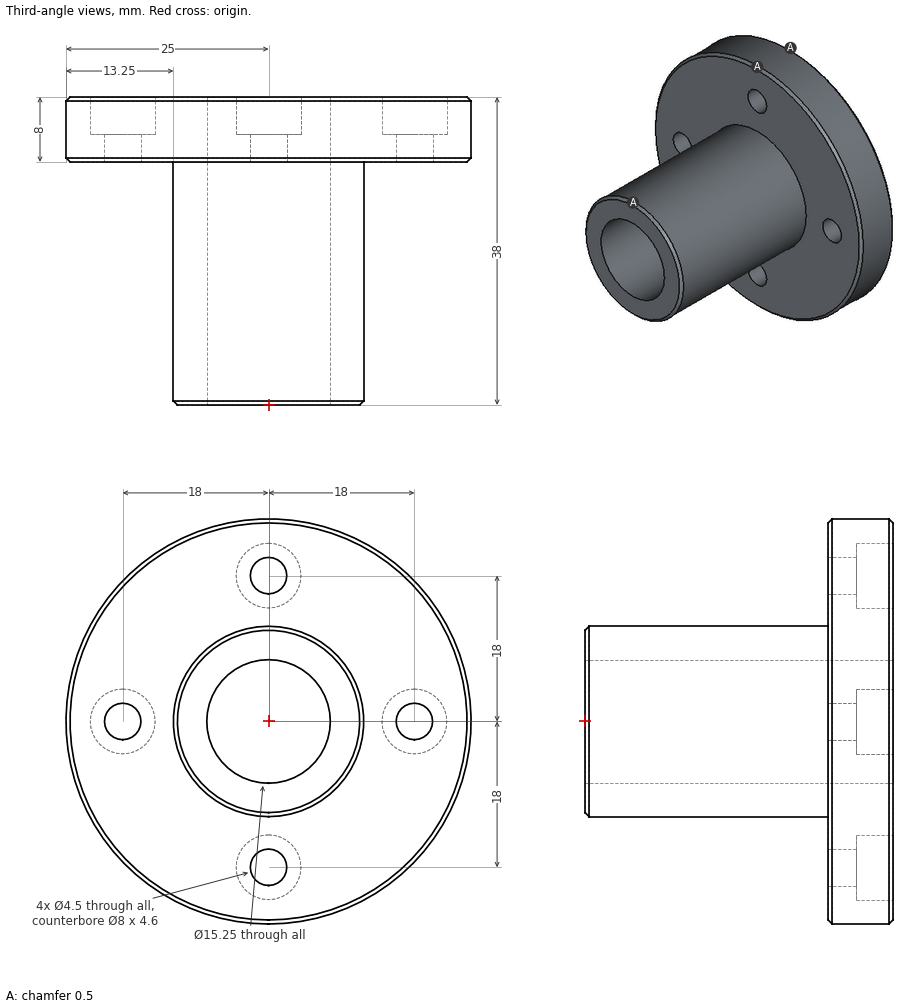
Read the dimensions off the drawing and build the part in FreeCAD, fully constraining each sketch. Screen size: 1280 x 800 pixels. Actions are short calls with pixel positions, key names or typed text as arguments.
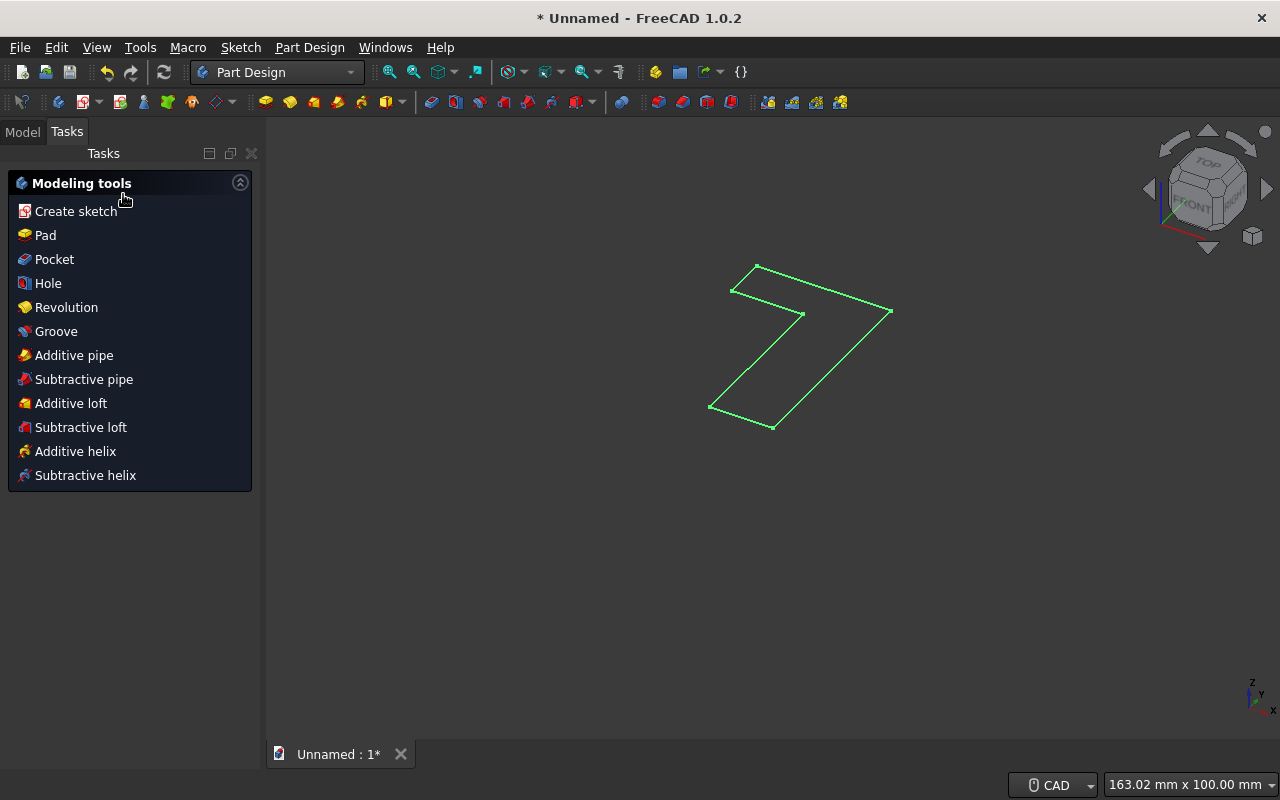
click(290, 102)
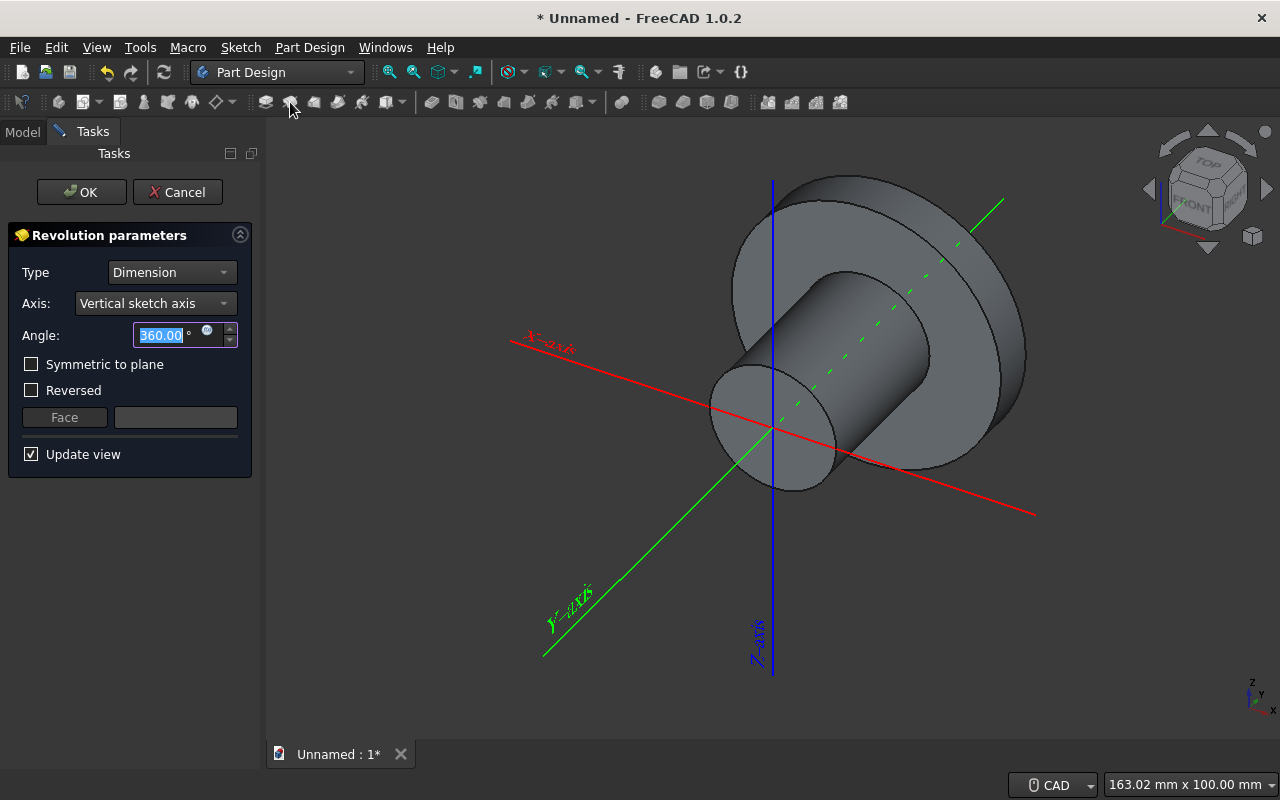
click(82, 192)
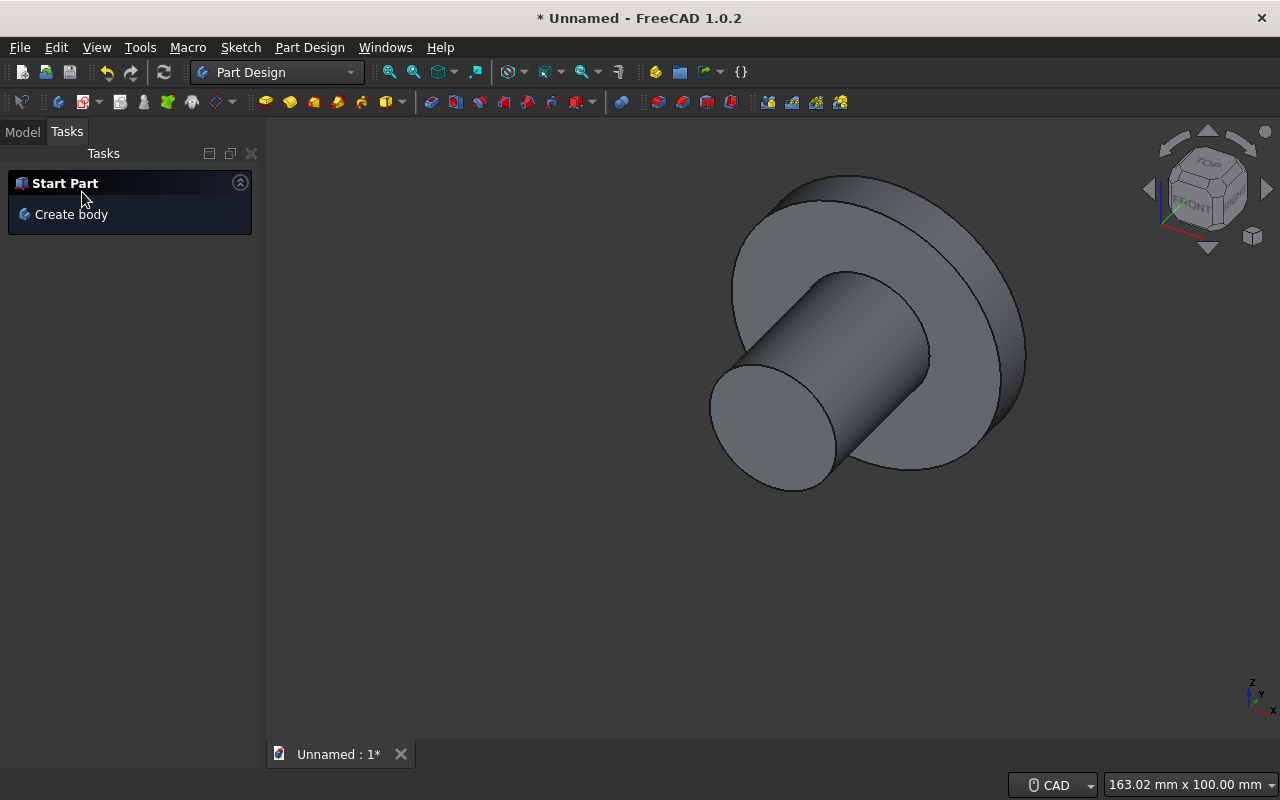
key(4)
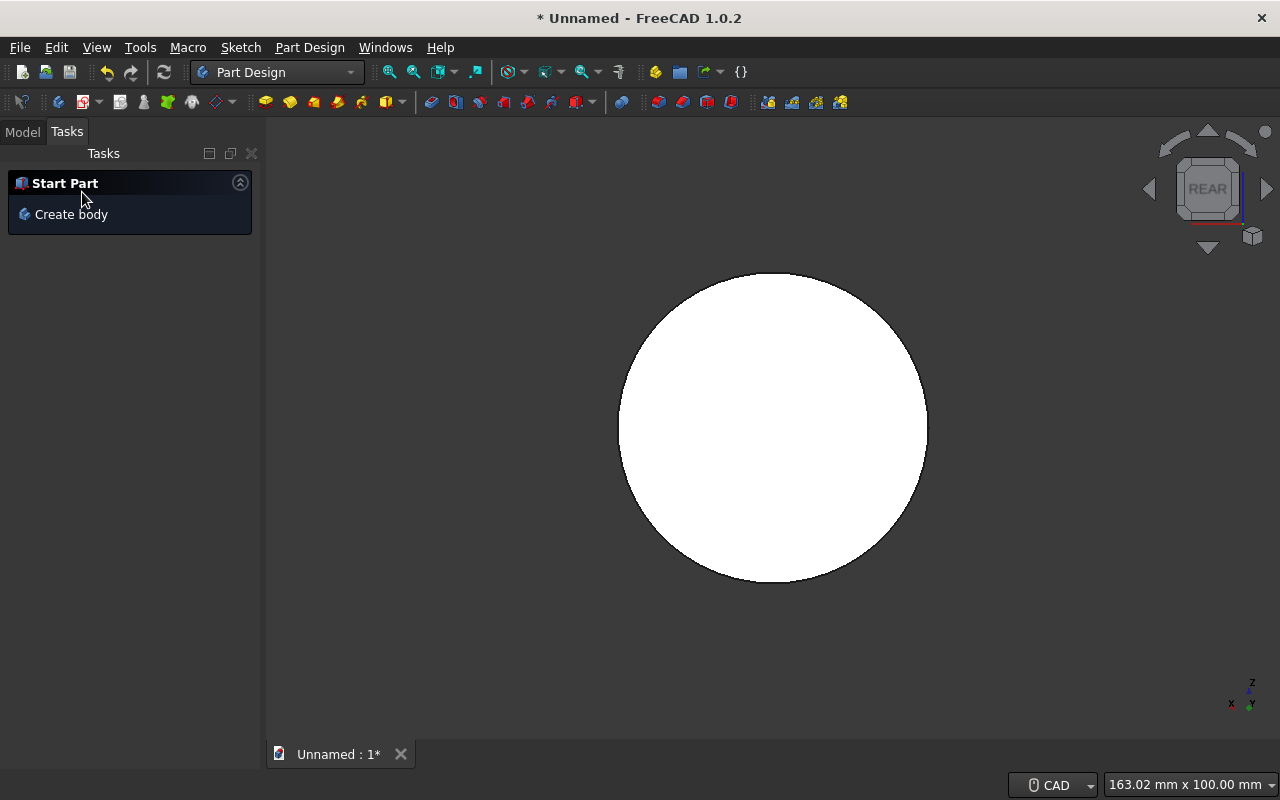
click(773, 427)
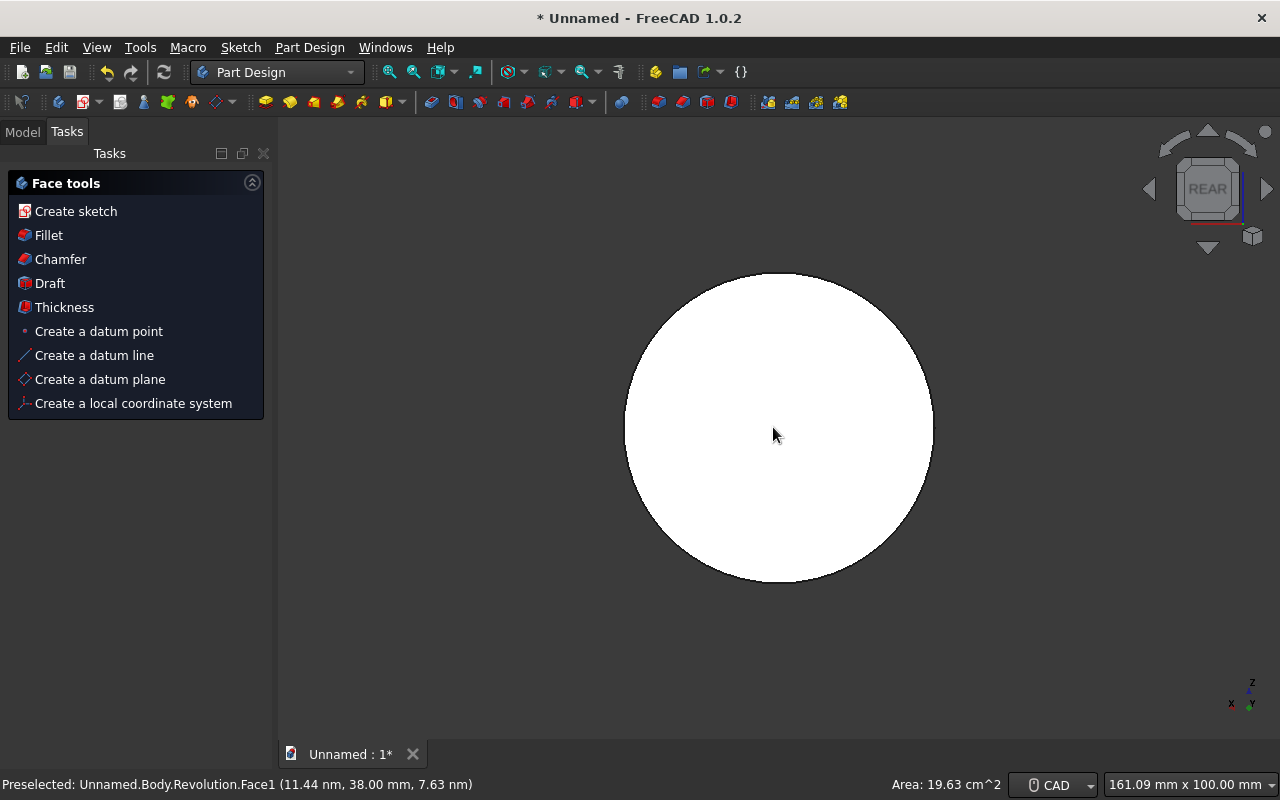
click(84, 102)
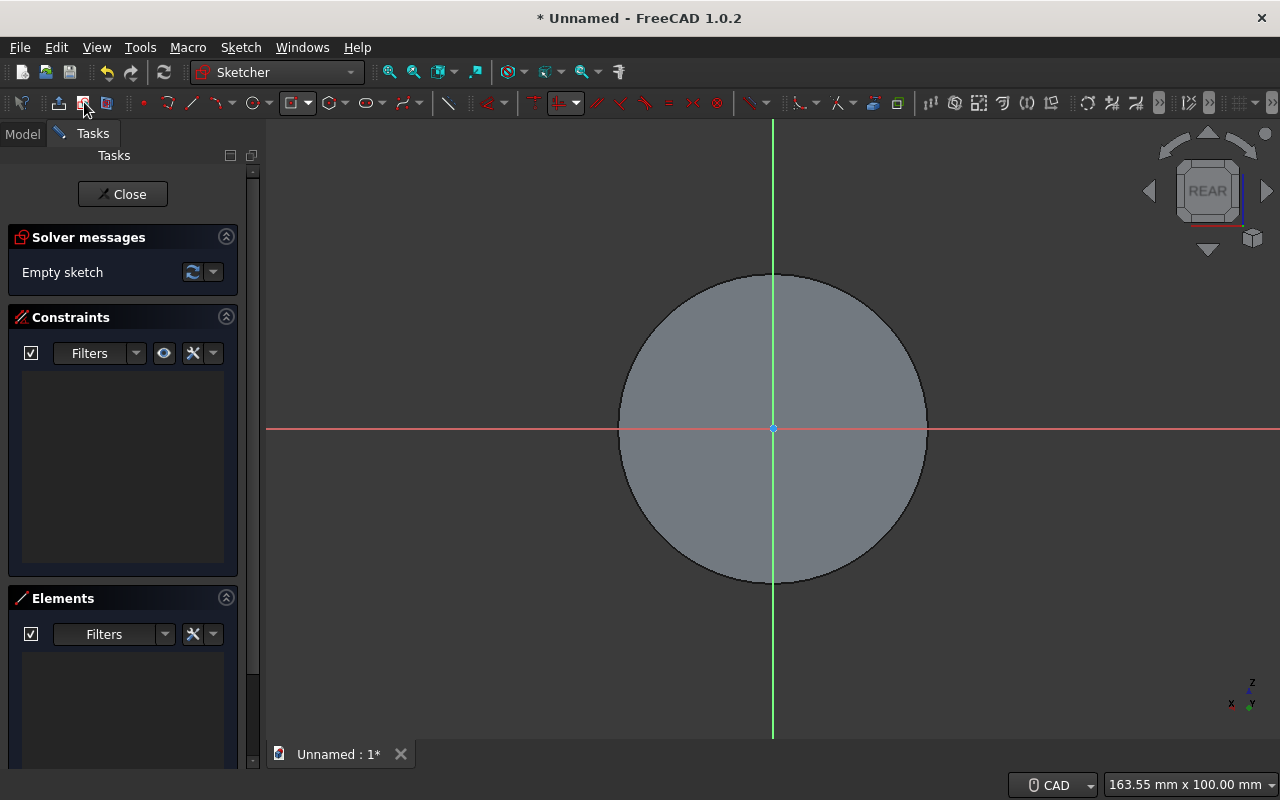
scroll(795, 429, up, 7)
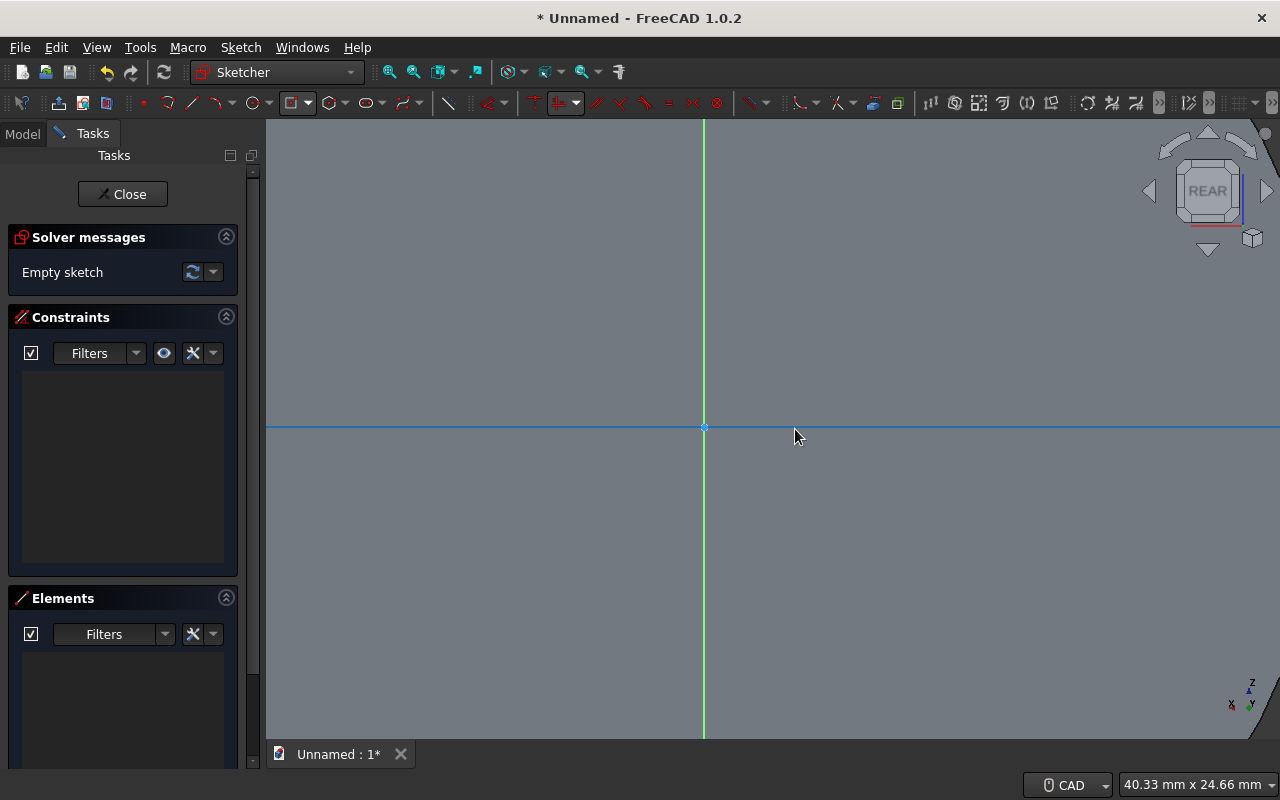
click(254, 104)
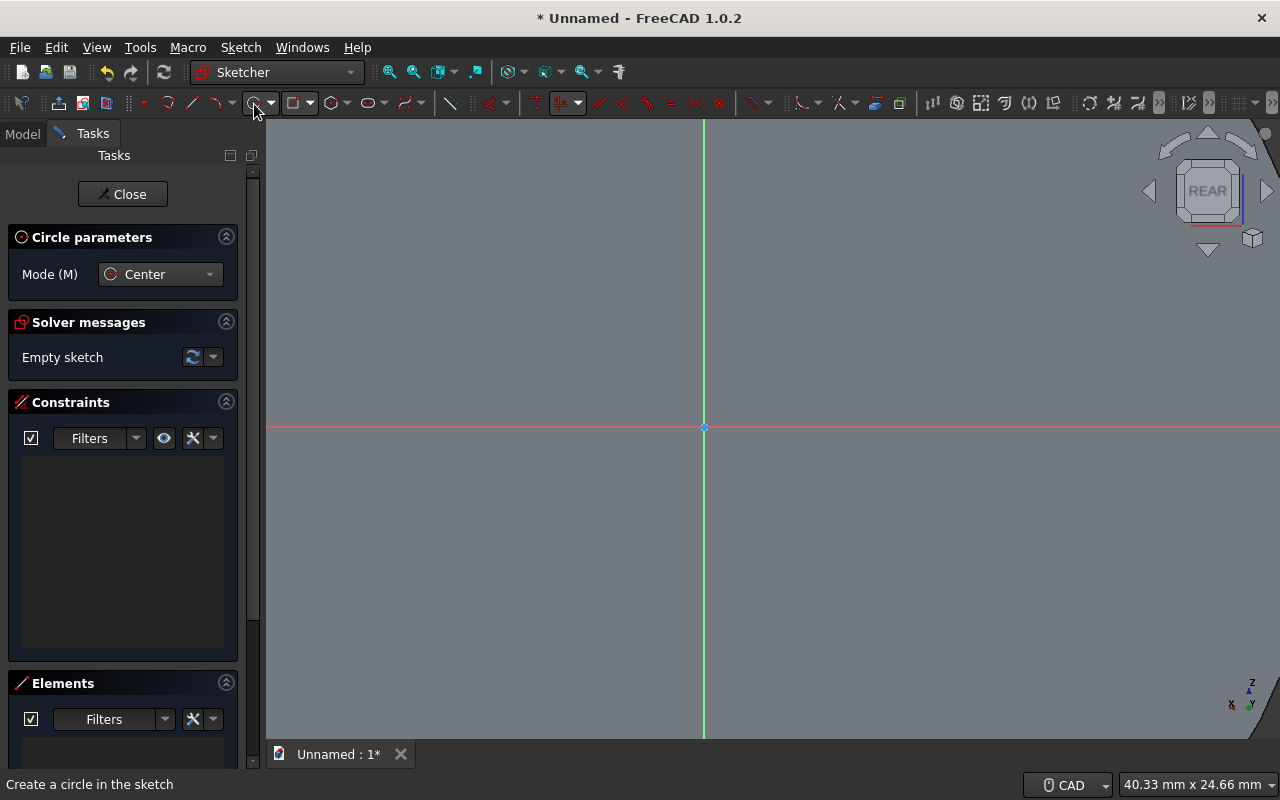
click(704, 427)
click(840, 292)
key(Escape)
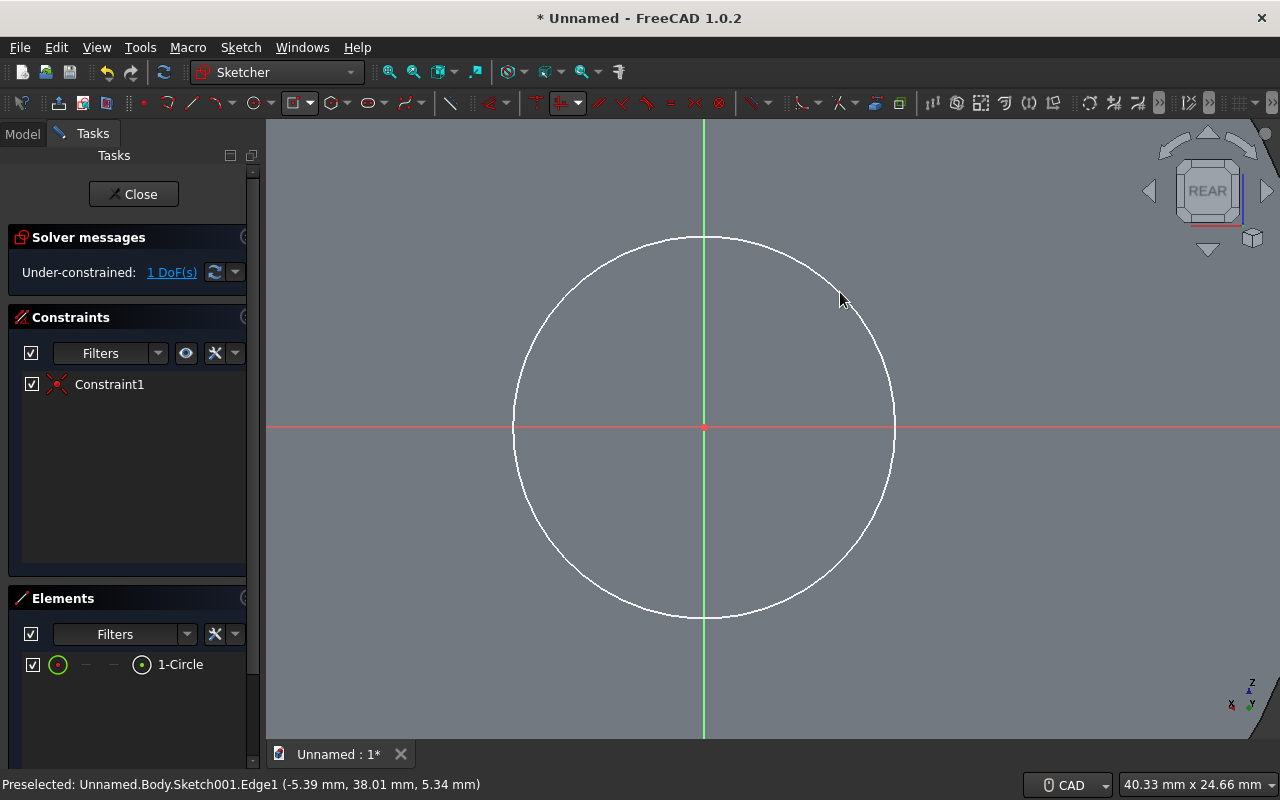
click(490, 104)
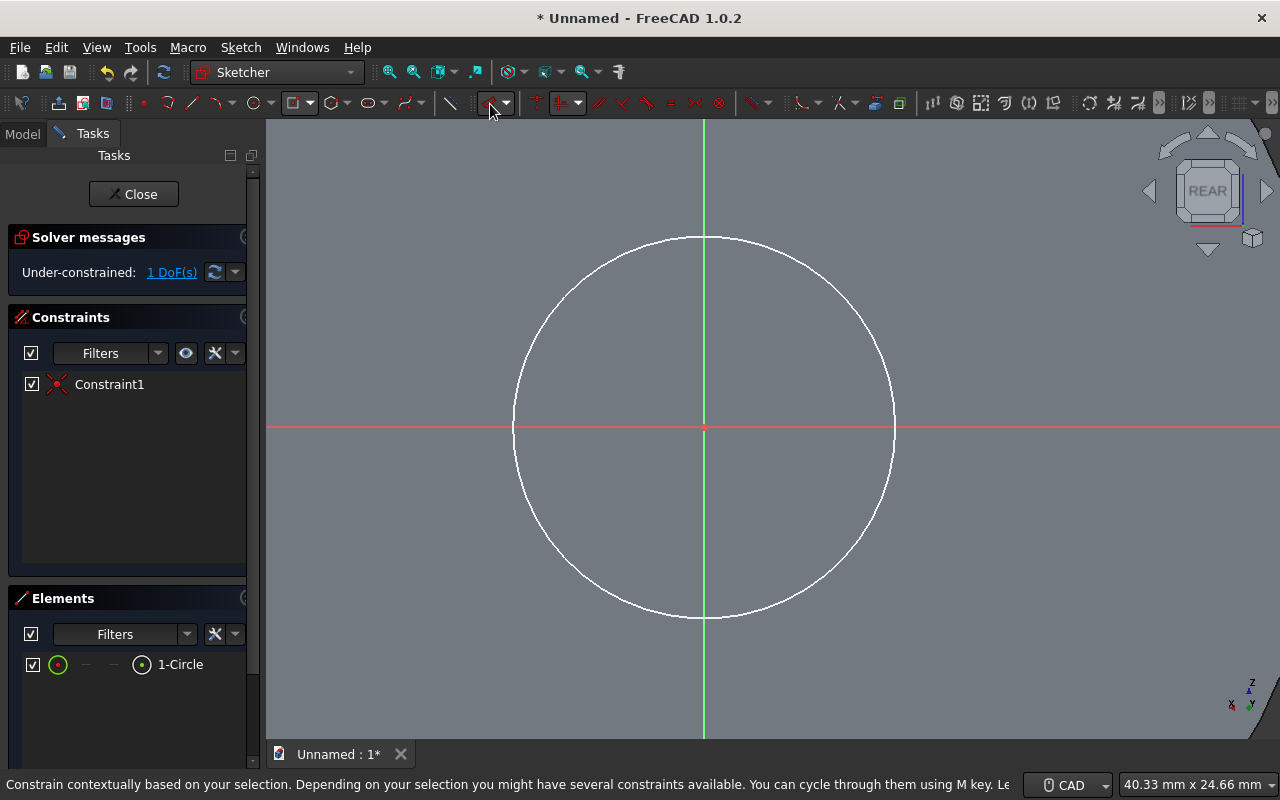
click(839, 292)
click(862, 269)